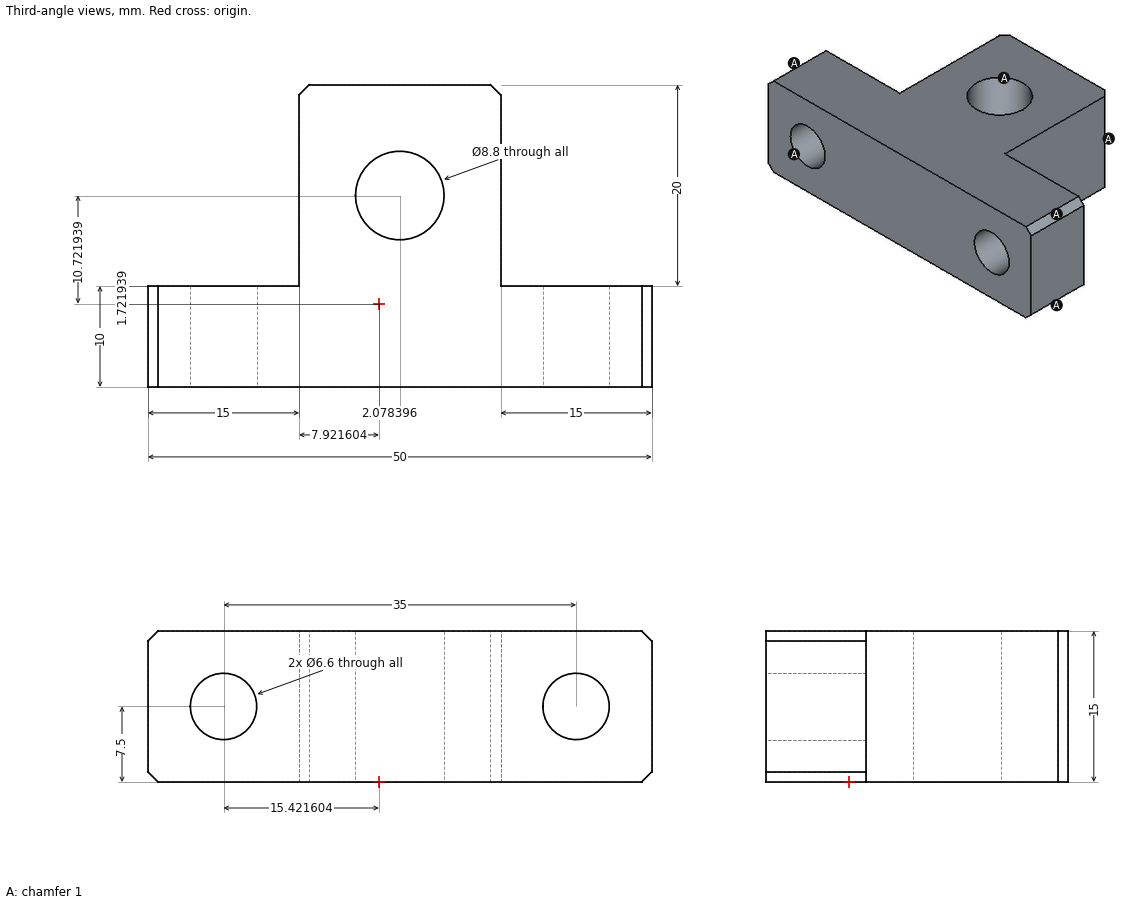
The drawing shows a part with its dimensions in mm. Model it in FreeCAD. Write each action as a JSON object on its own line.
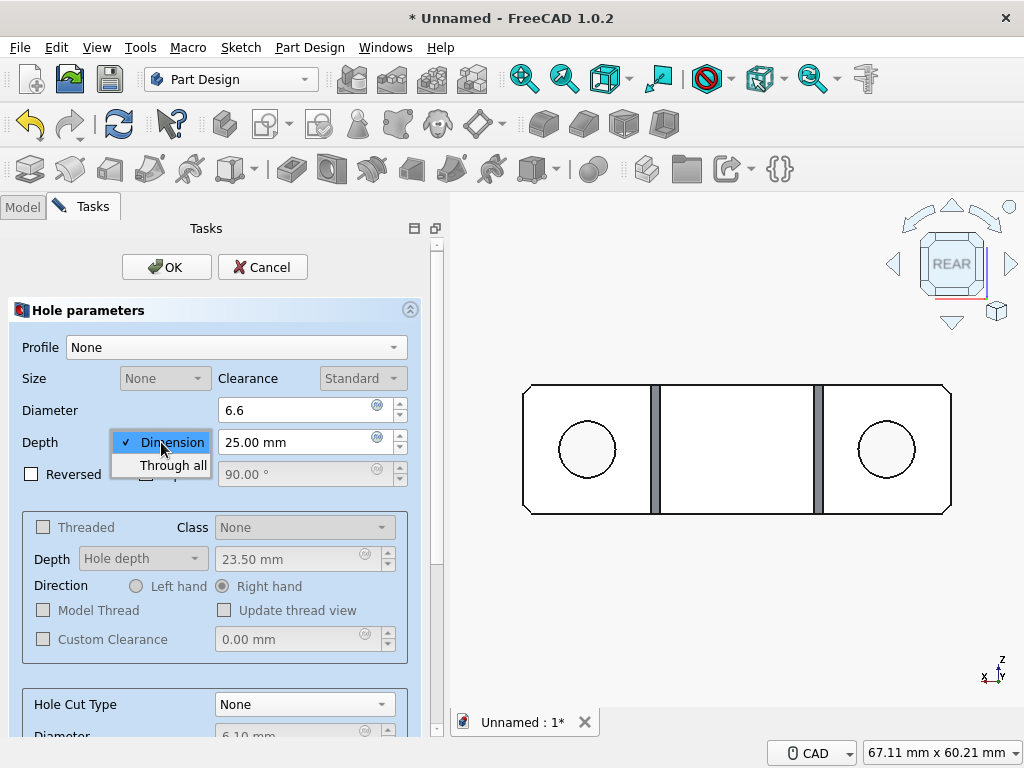
{"action": "left_click", "coordinate": [160, 466]}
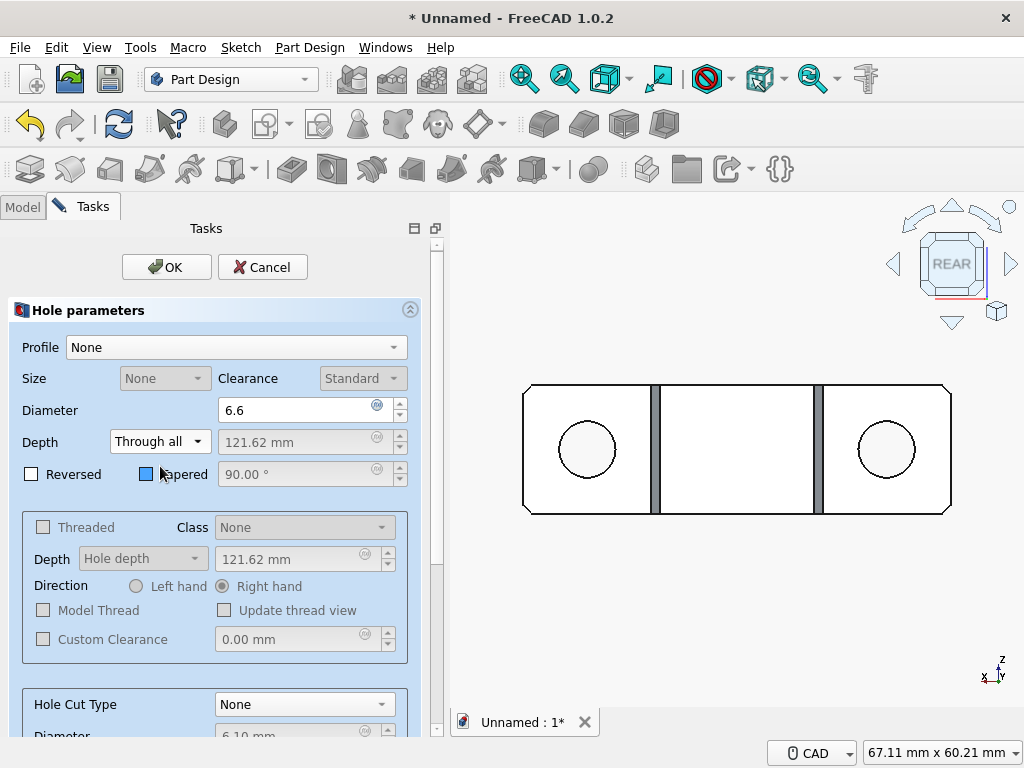
{"action": "left_click", "coordinate": [167, 267]}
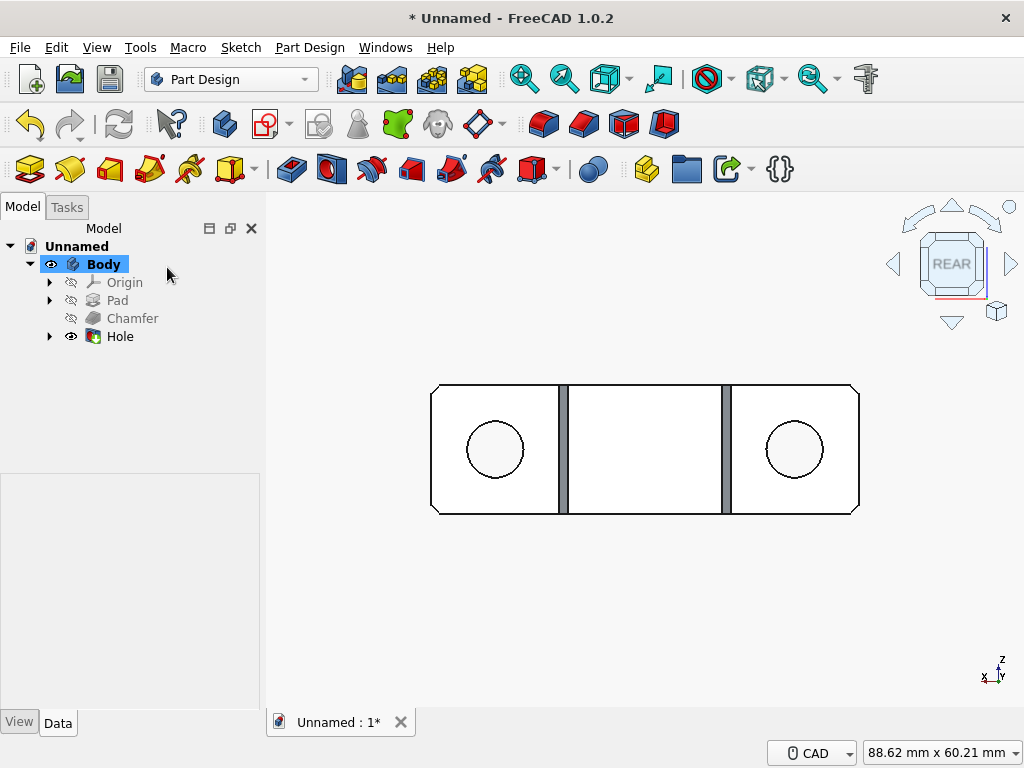
{"action": "key", "text": "0"}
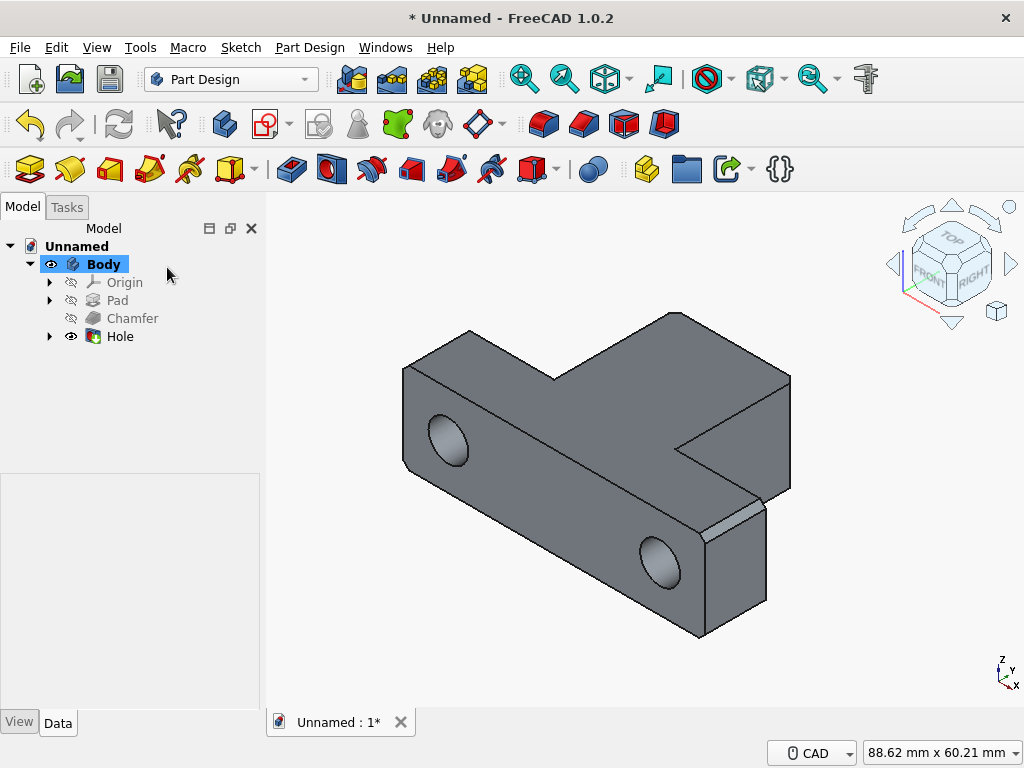
{"action": "left_click", "coordinate": [671, 381]}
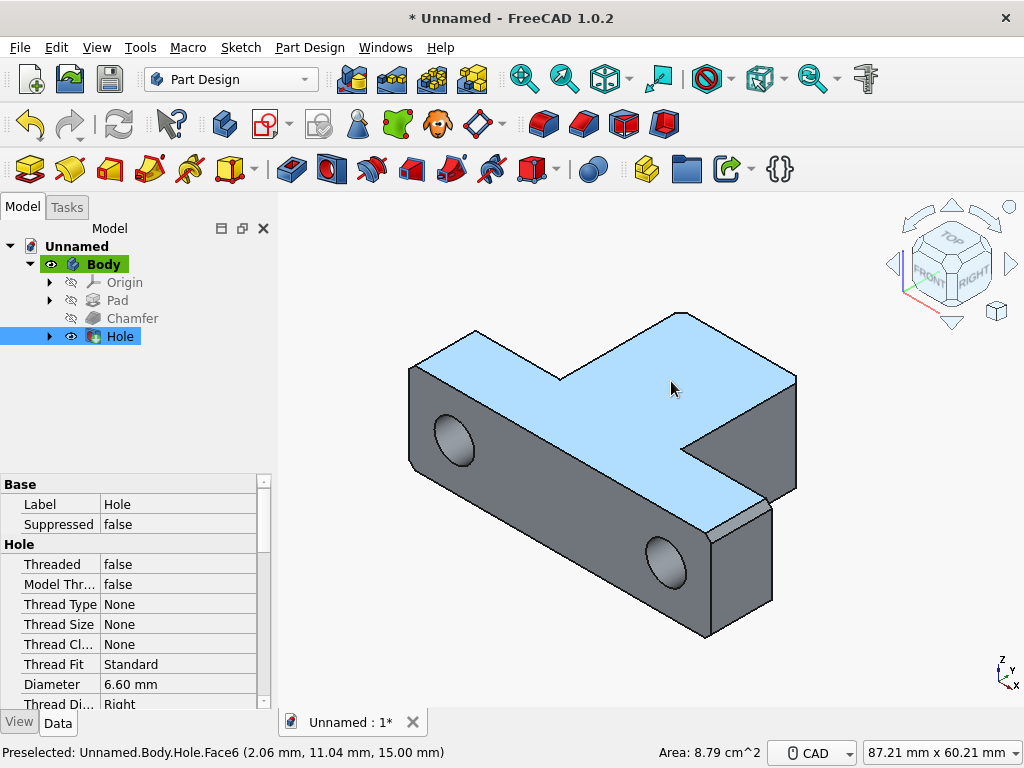
{"action": "left_click", "coordinate": [266, 124]}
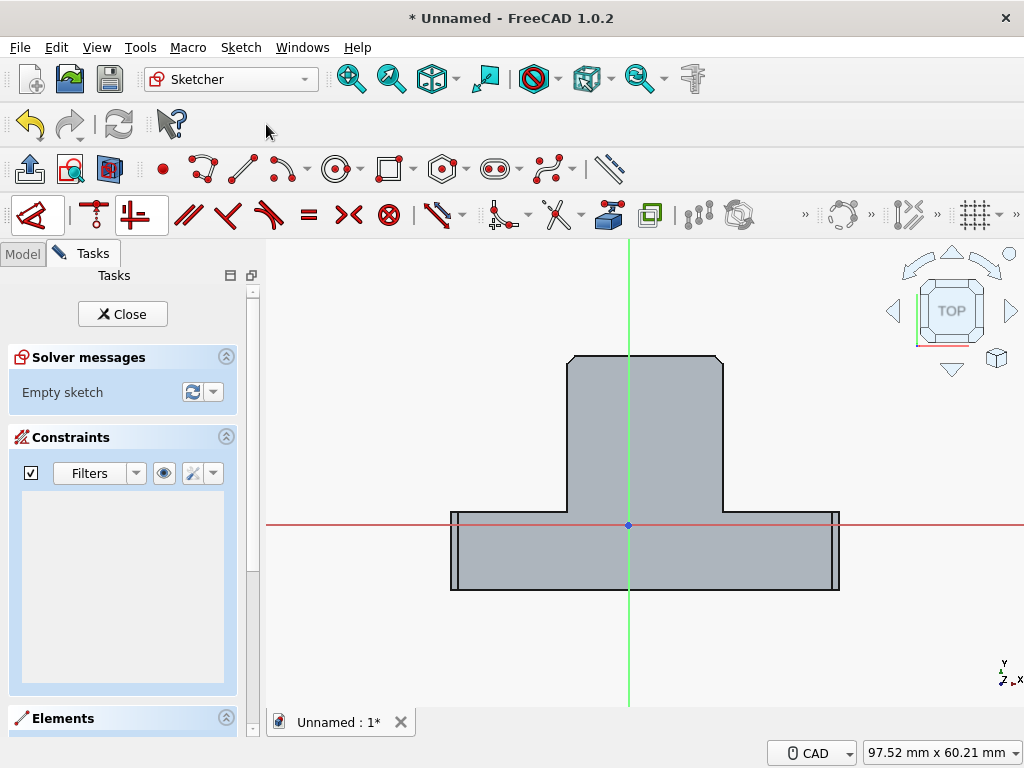
{"action": "scroll", "coordinate": [685, 463], "scroll_direction": "up", "scroll_amount": 5}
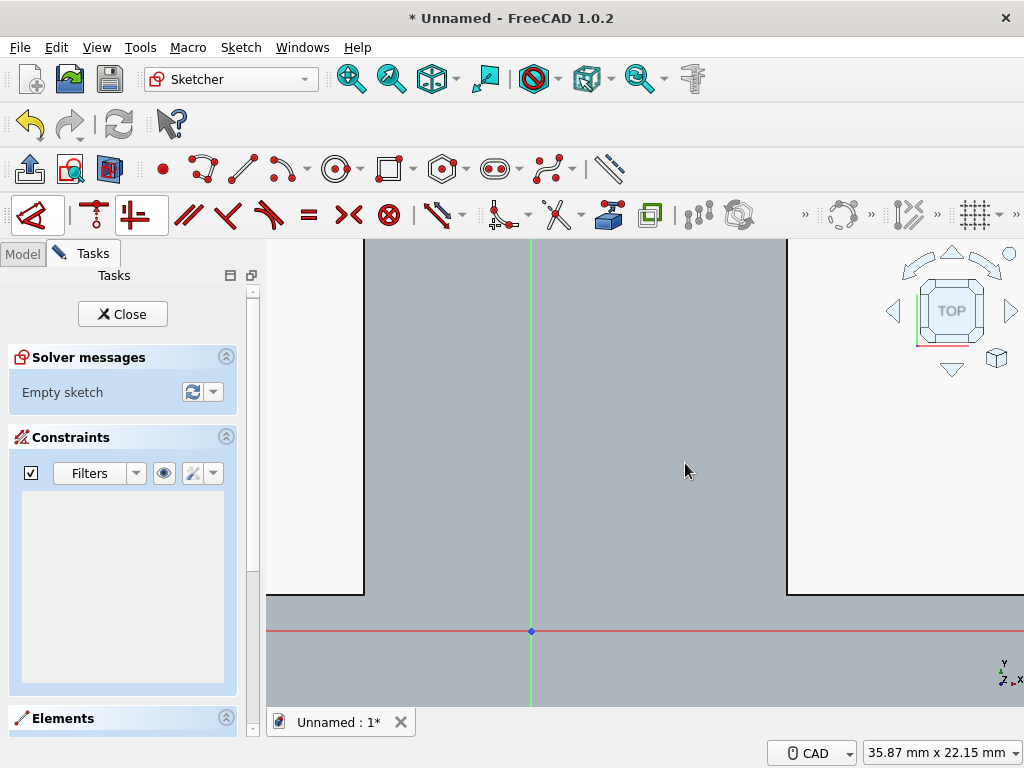
{"action": "left_click", "coordinate": [336, 170]}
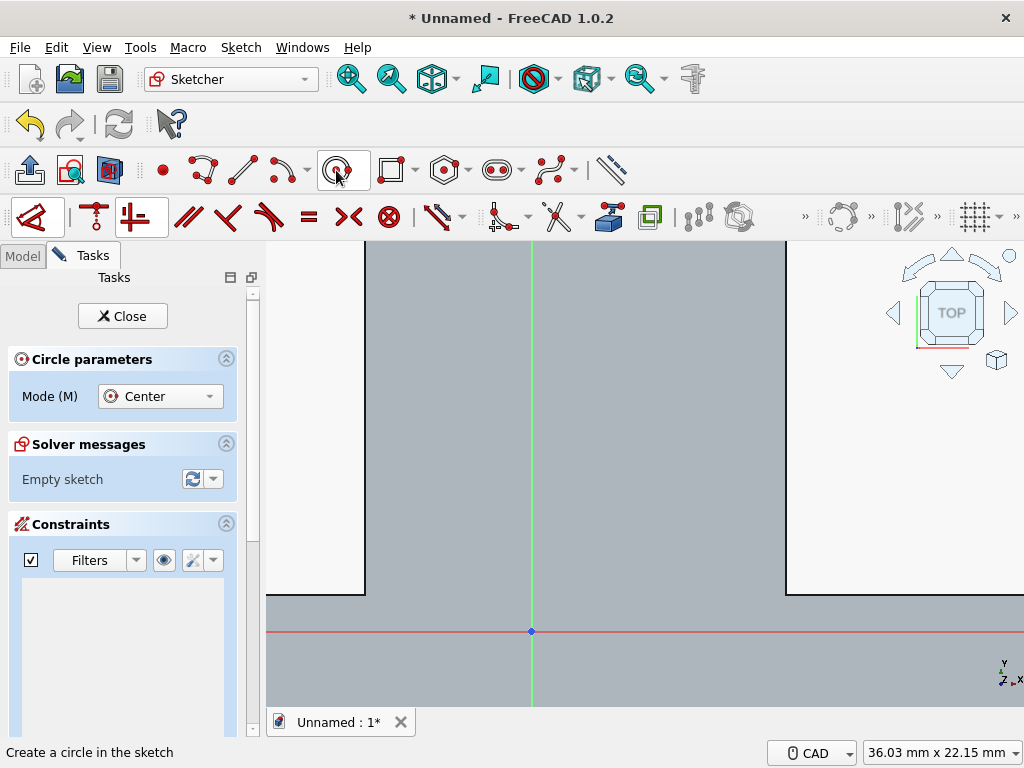
{"action": "left_click", "coordinate": [576, 406]}
{"action": "mouse_move", "coordinate": [641, 341]}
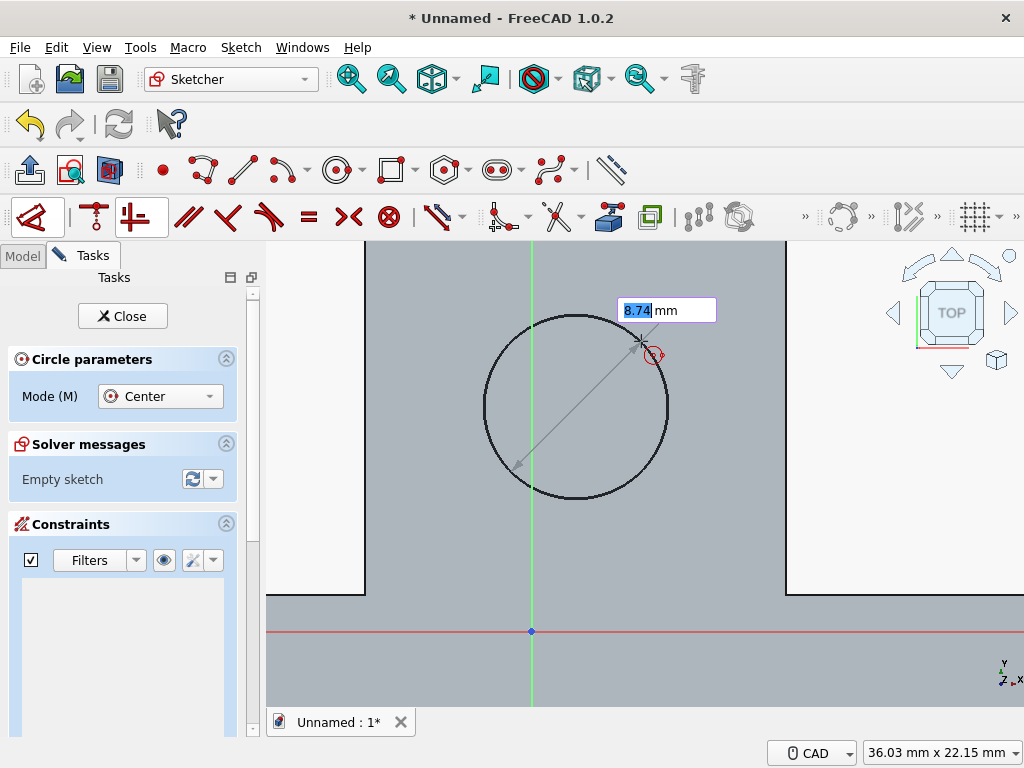
{"action": "type", "text": "8.8"}
{"action": "key", "text": "Return"}
{"action": "key", "text": "Escape"}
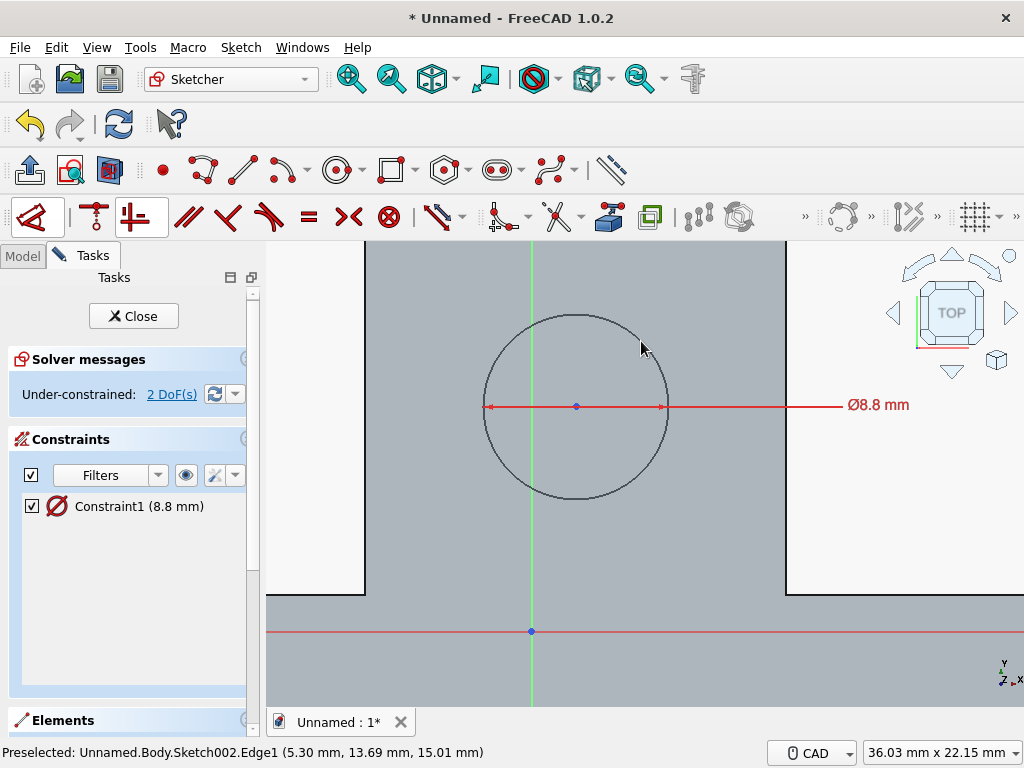
{"action": "left_click", "coordinate": [576, 407]}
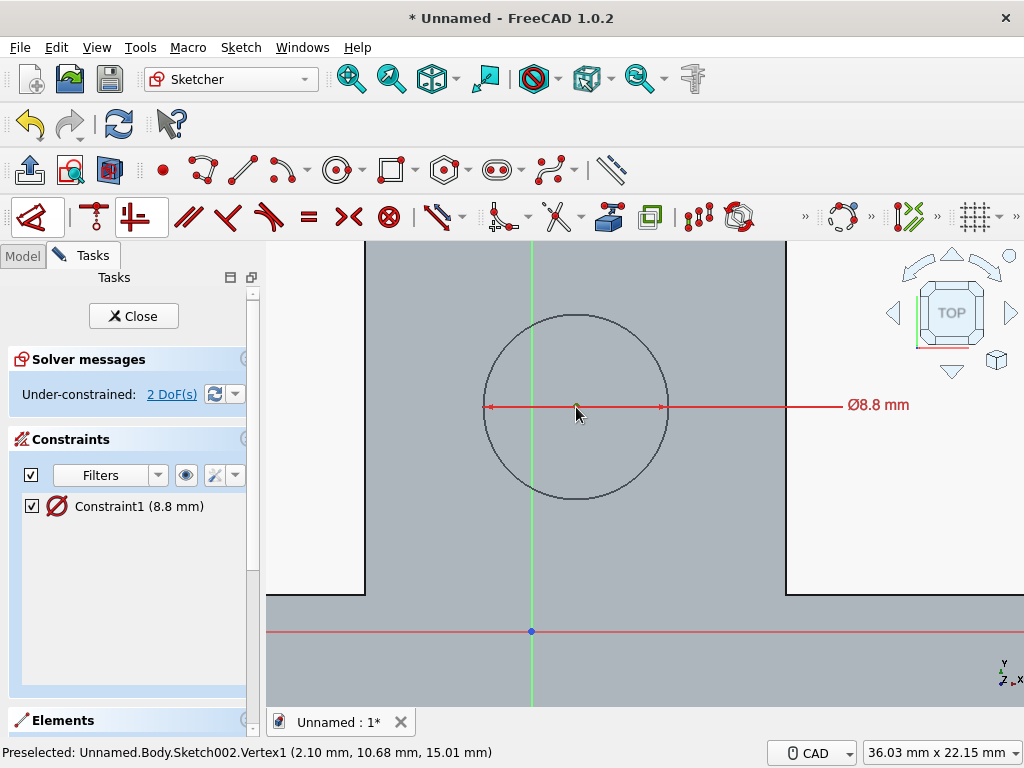
{"action": "key", "text": "l"}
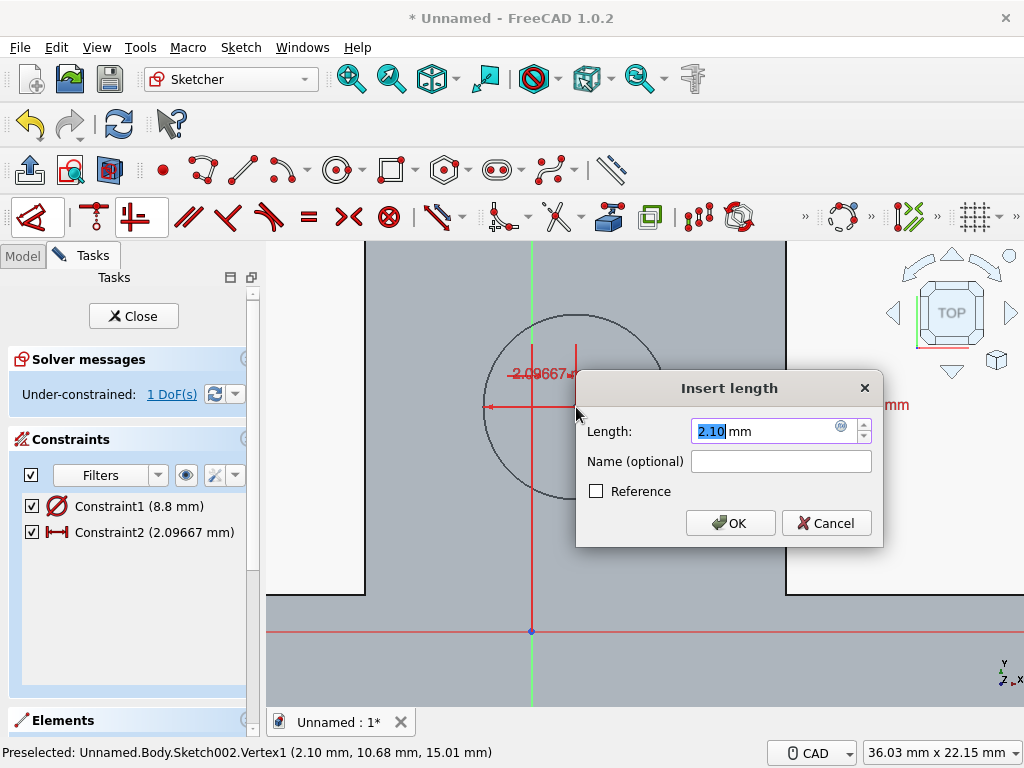
{"action": "type", "text": "2.078396"}
{"action": "key", "text": "Return"}